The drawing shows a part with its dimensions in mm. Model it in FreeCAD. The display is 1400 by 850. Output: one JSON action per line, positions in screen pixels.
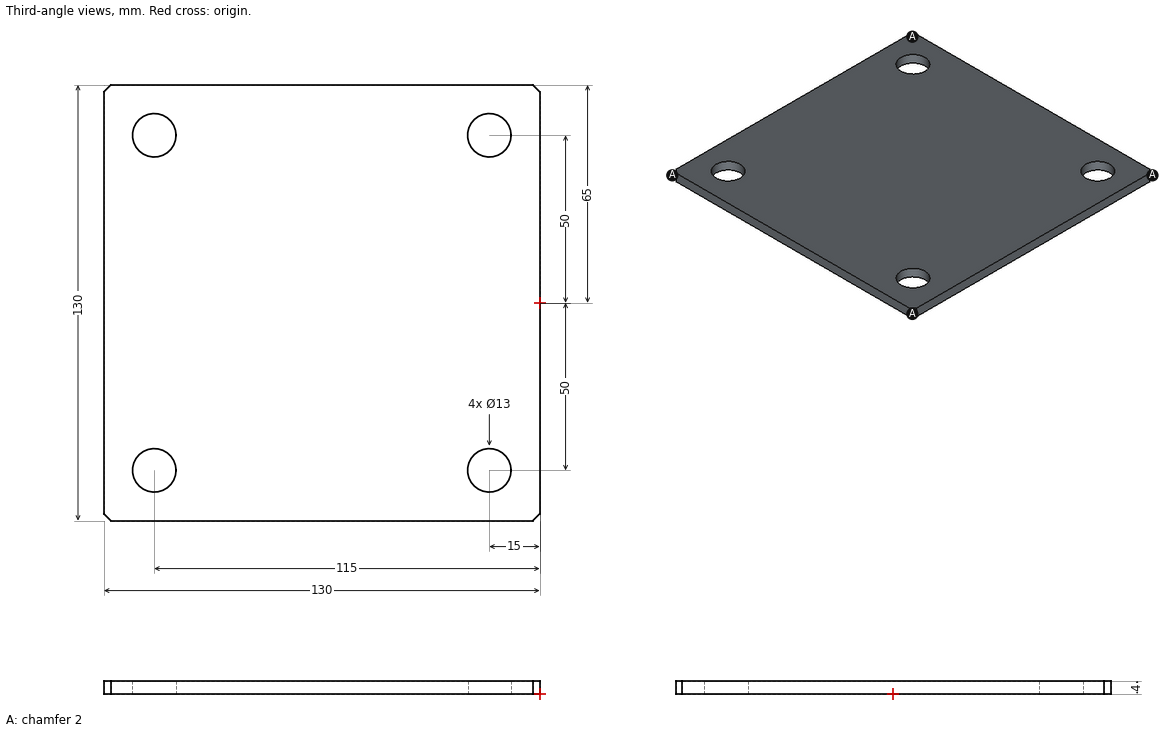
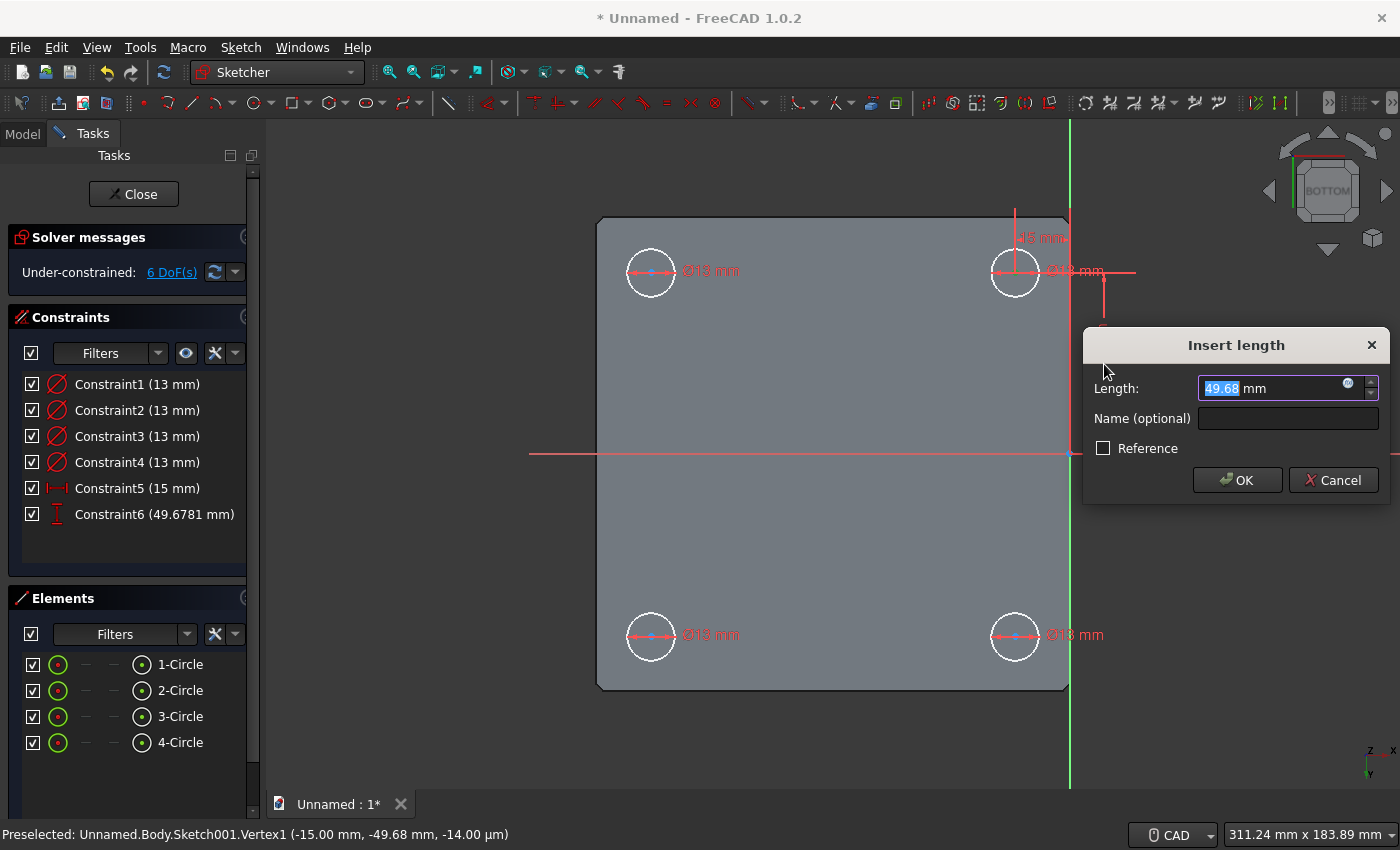
{"action": "type", "text": "50"}
{"action": "key", "text": "Return"}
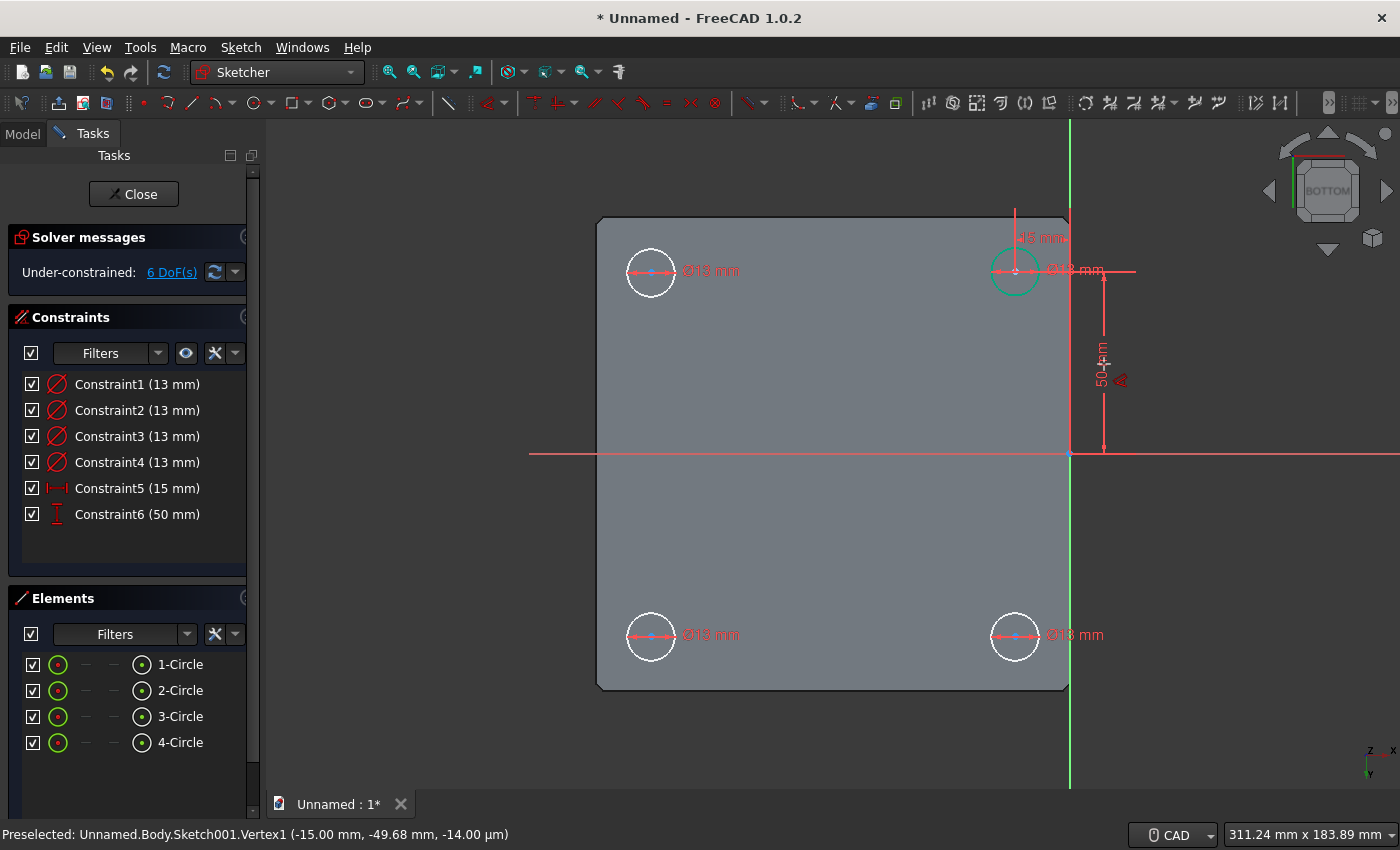
{"action": "left_click", "coordinate": [1015, 637]}
{"action": "left_click", "coordinate": [1042, 671]}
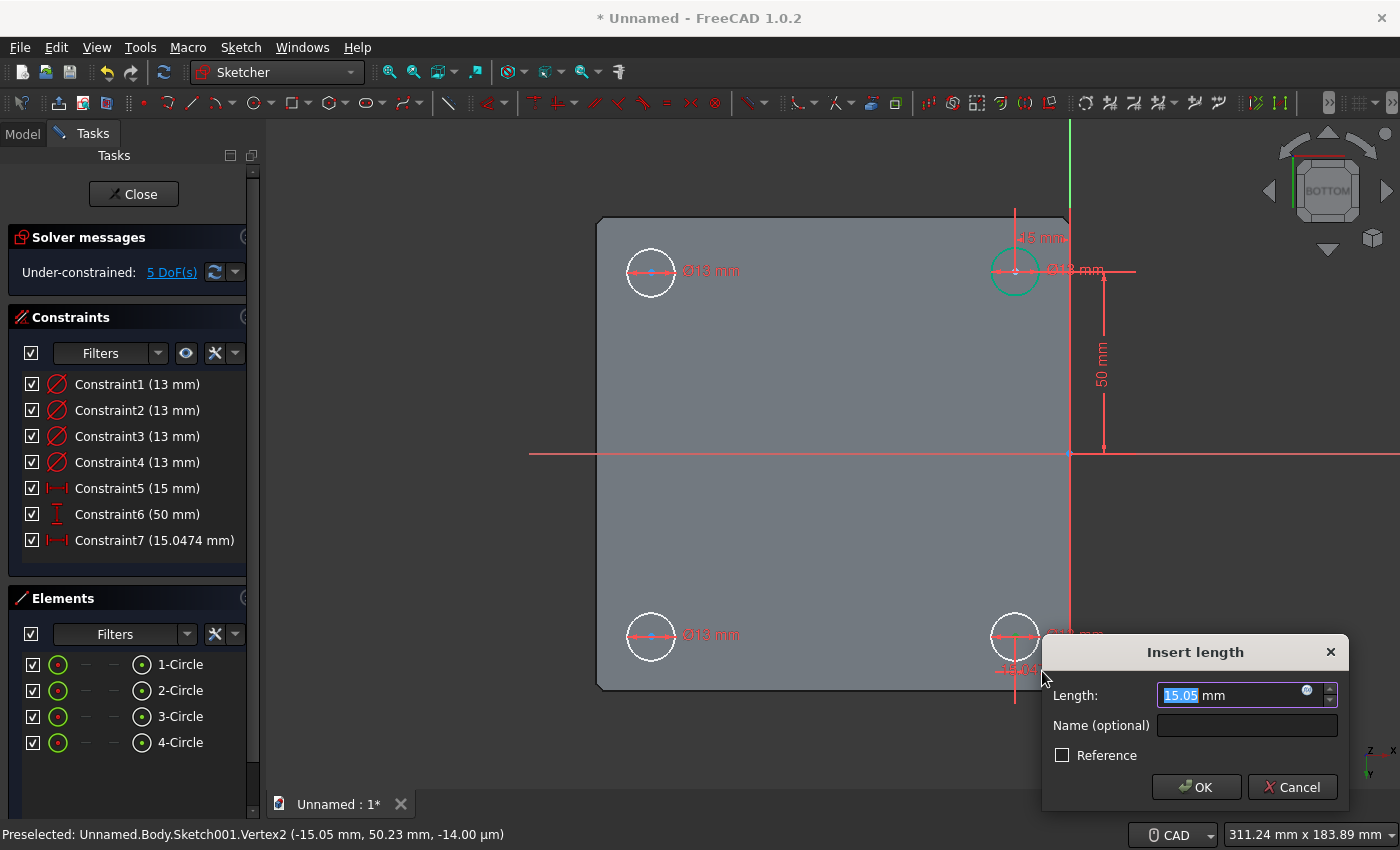
{"action": "type", "text": "15"}
{"action": "key", "text": "Return"}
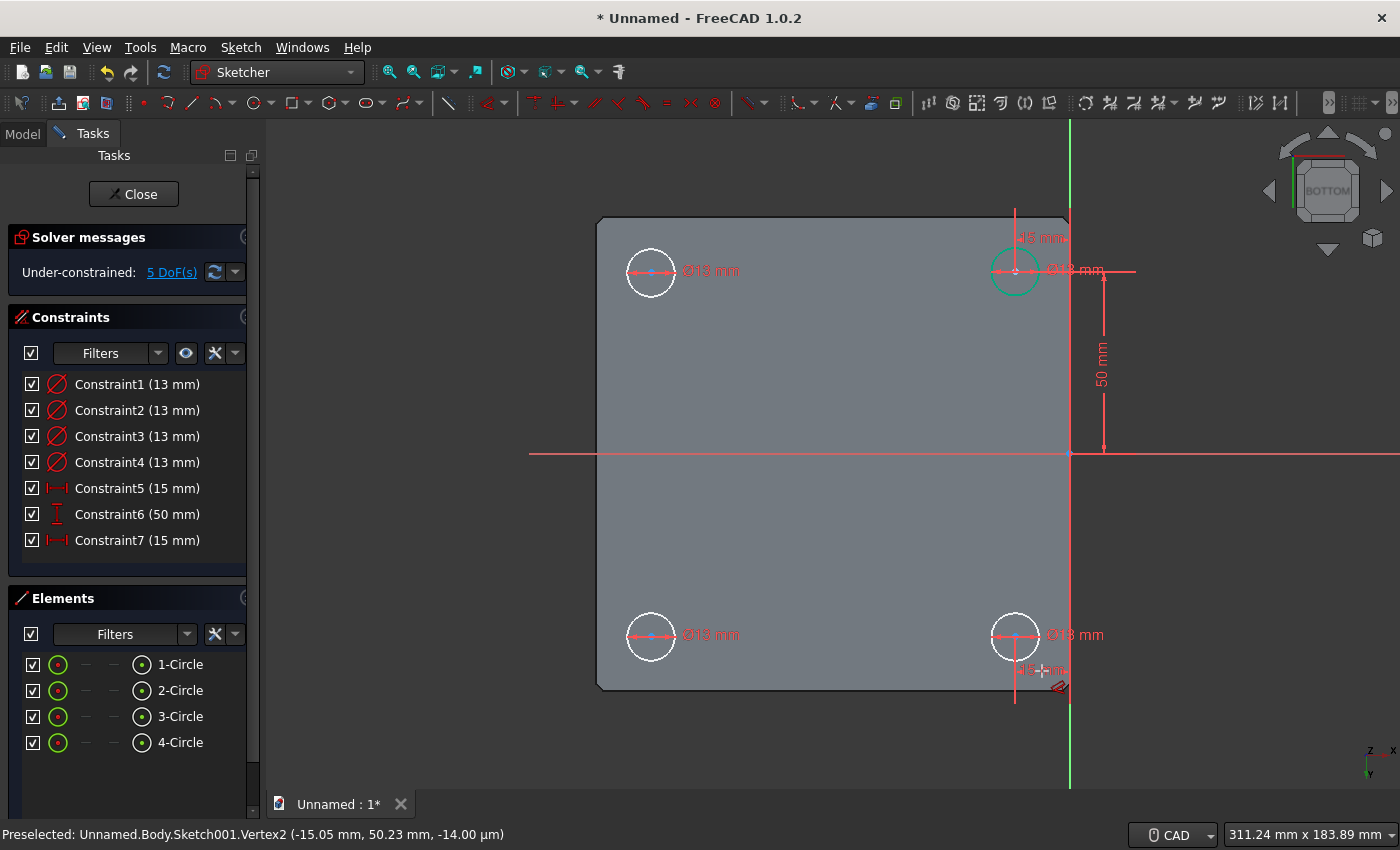
{"action": "left_click", "coordinate": [1015, 637]}
{"action": "left_click", "coordinate": [1104, 545]}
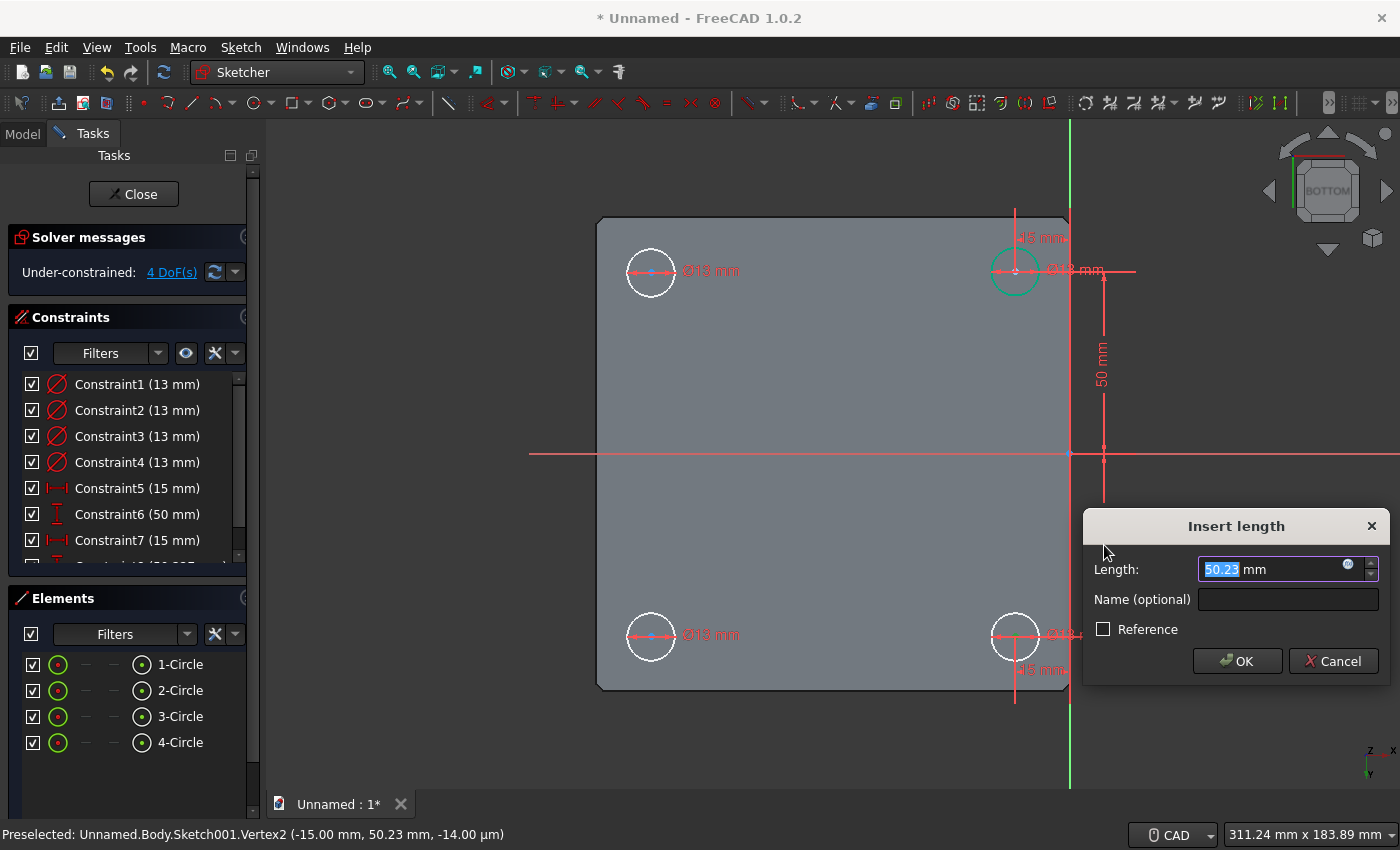
{"action": "type", "text": "50"}
{"action": "key", "text": "Return"}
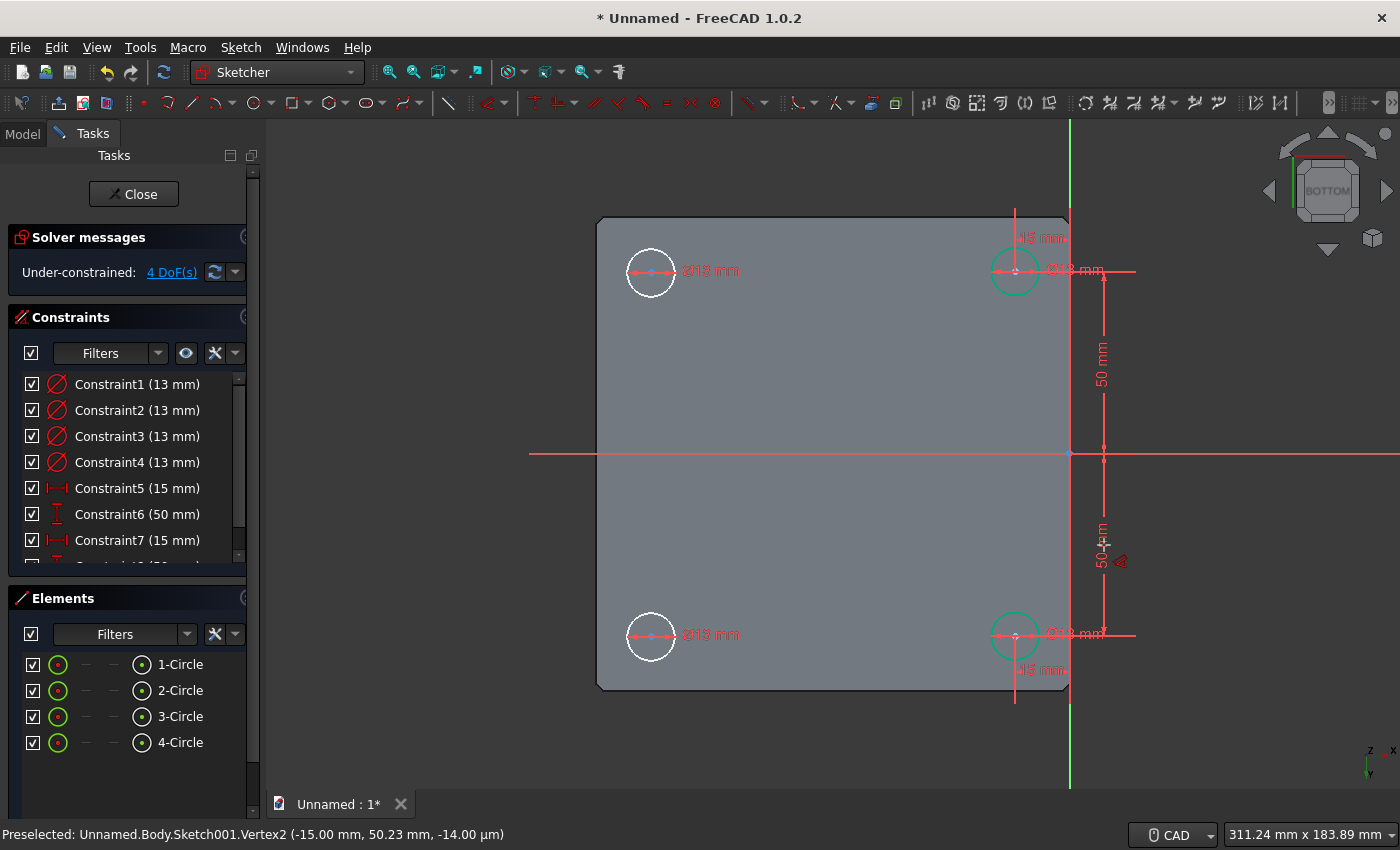
{"action": "left_click", "coordinate": [651, 273]}
{"action": "left_click", "coordinate": [1104, 322]}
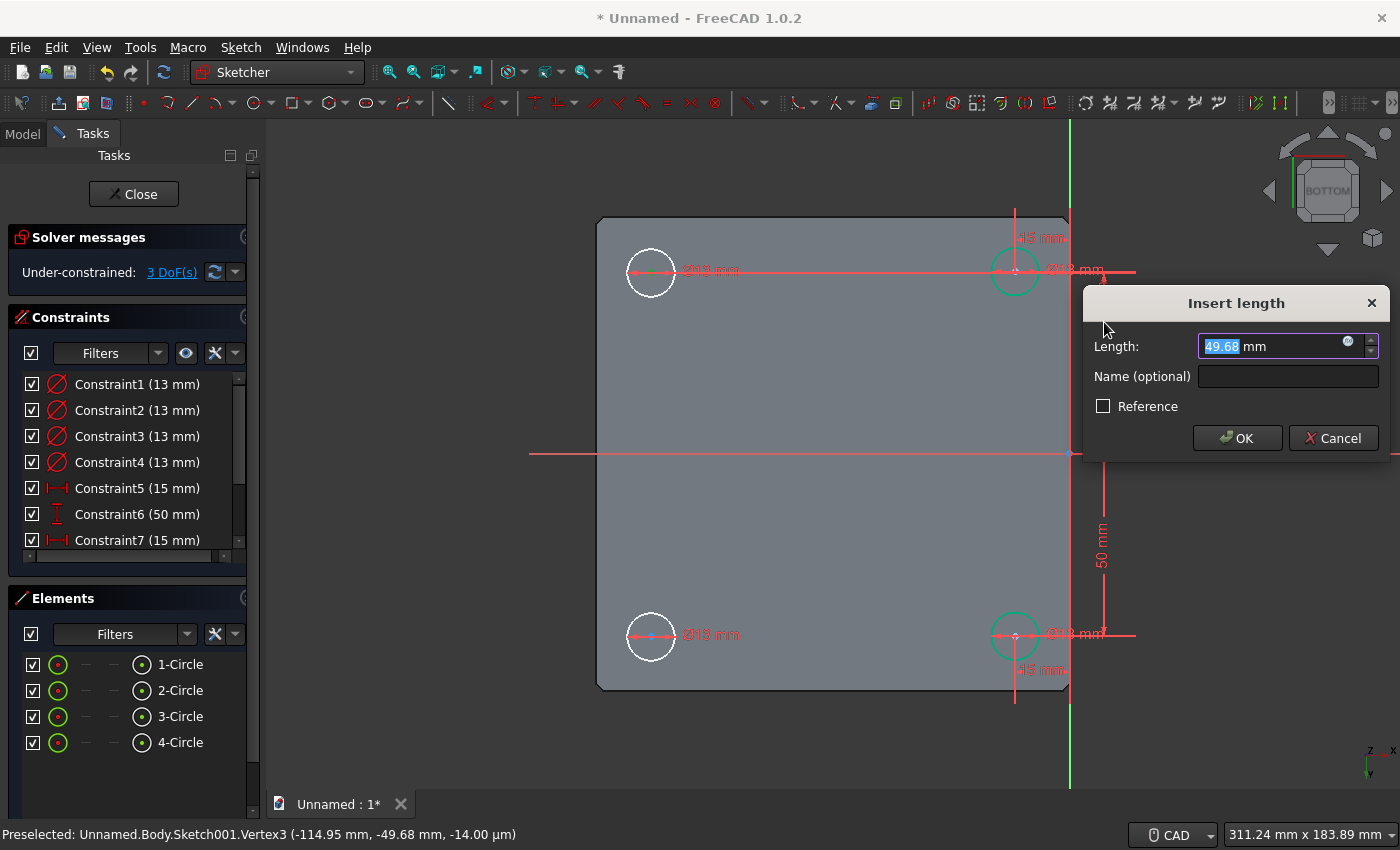
{"action": "type", "text": "50"}
{"action": "key", "text": "Return"}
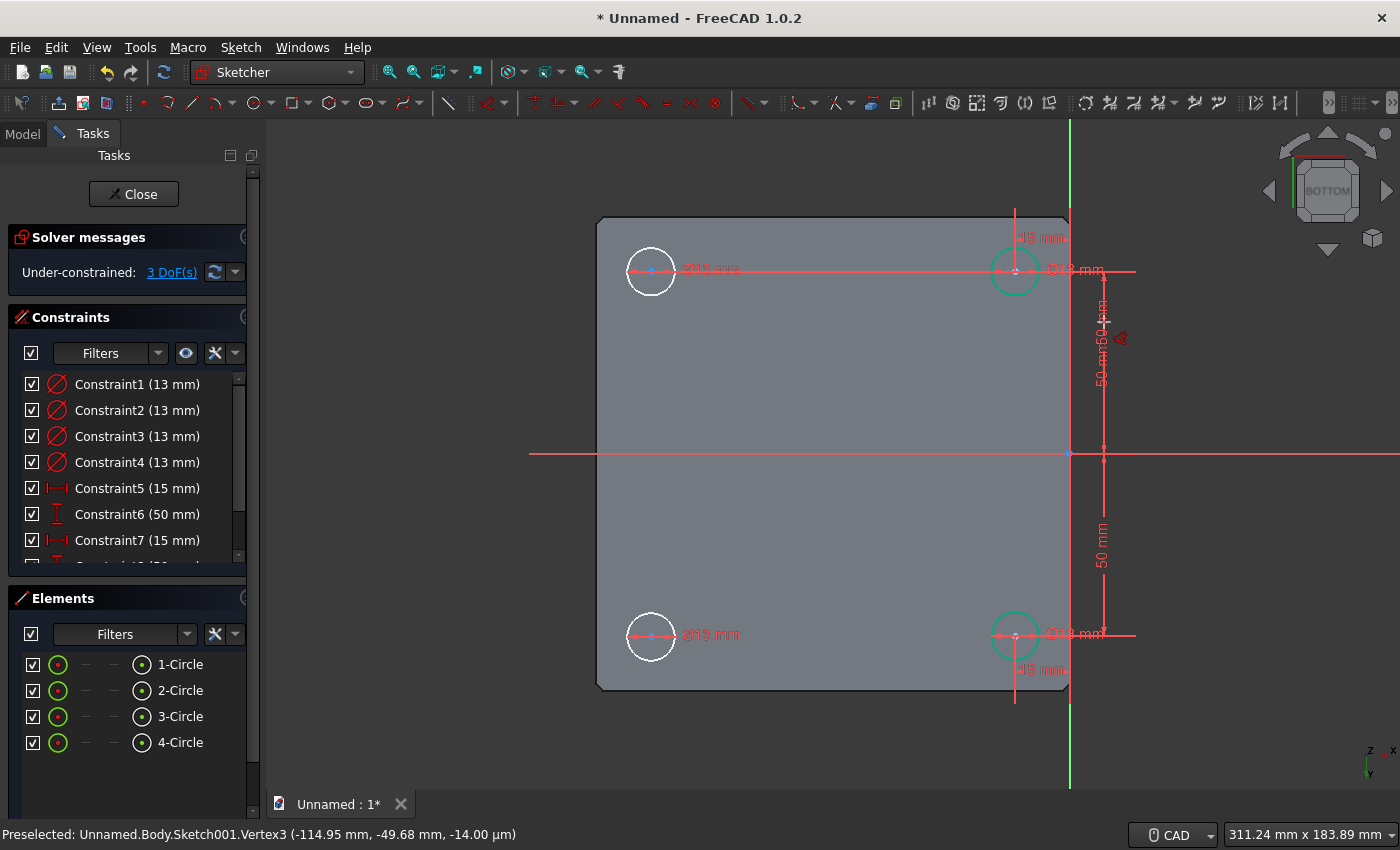
{"action": "left_click", "coordinate": [651, 637]}
{"action": "left_click", "coordinate": [1104, 503]}